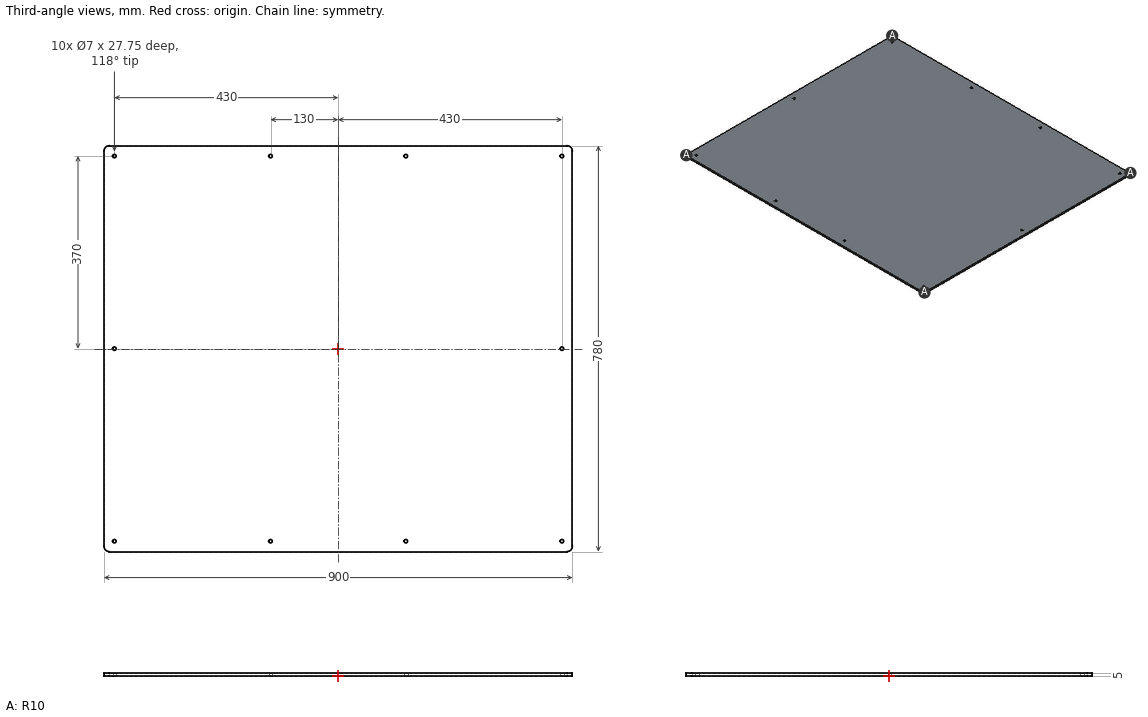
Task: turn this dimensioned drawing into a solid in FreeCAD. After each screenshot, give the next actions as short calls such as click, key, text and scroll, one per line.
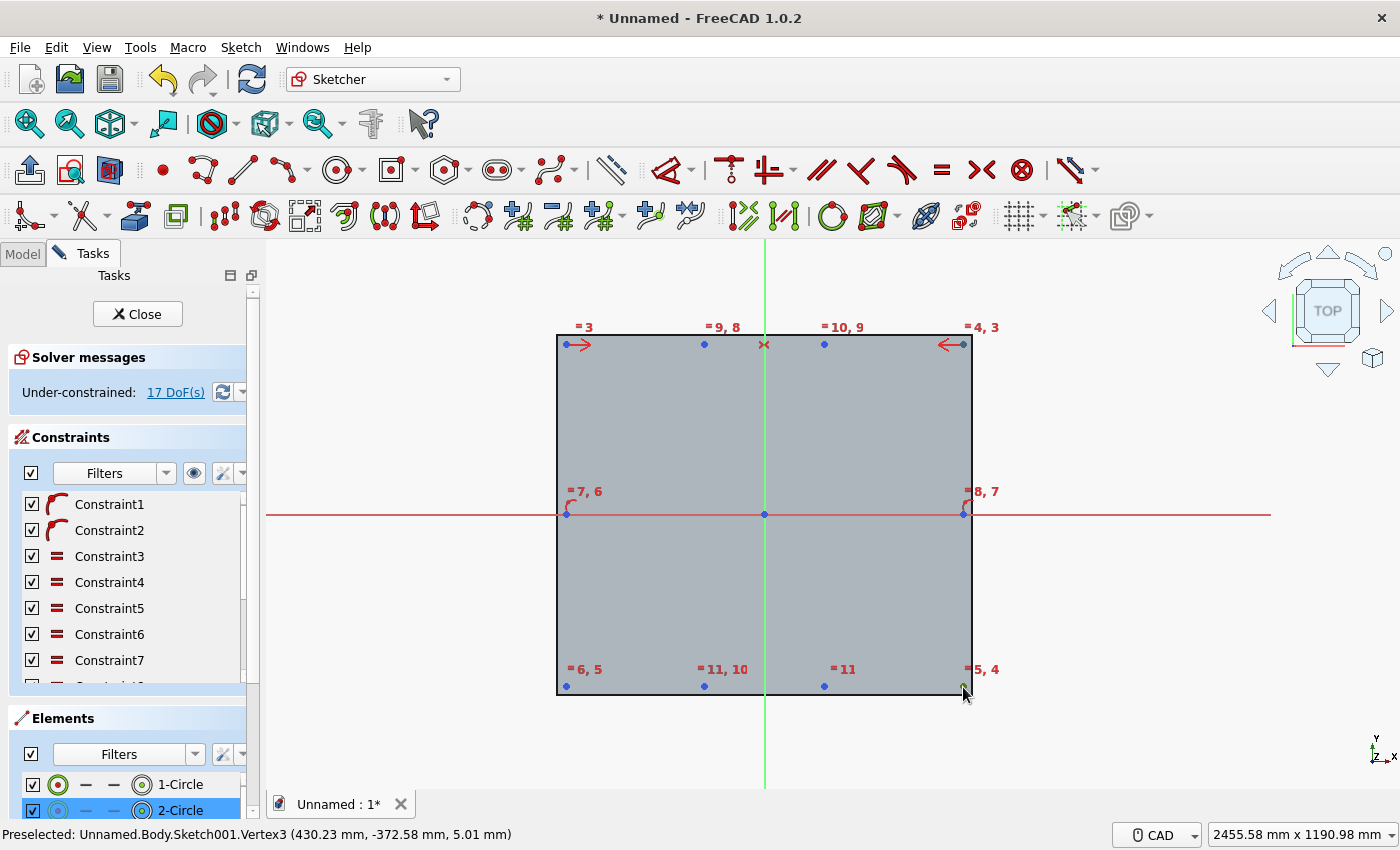
click(361, 515)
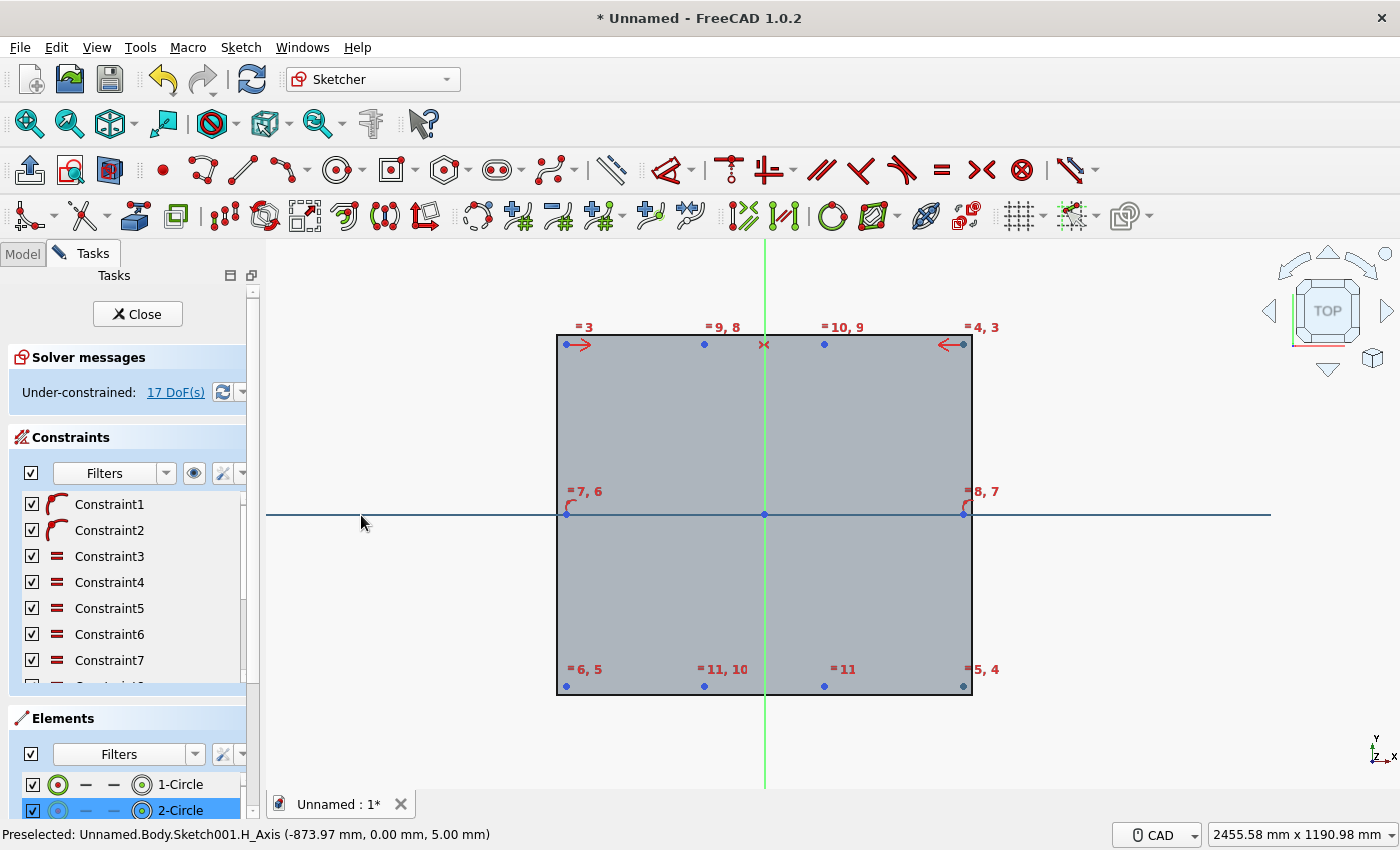
key(s)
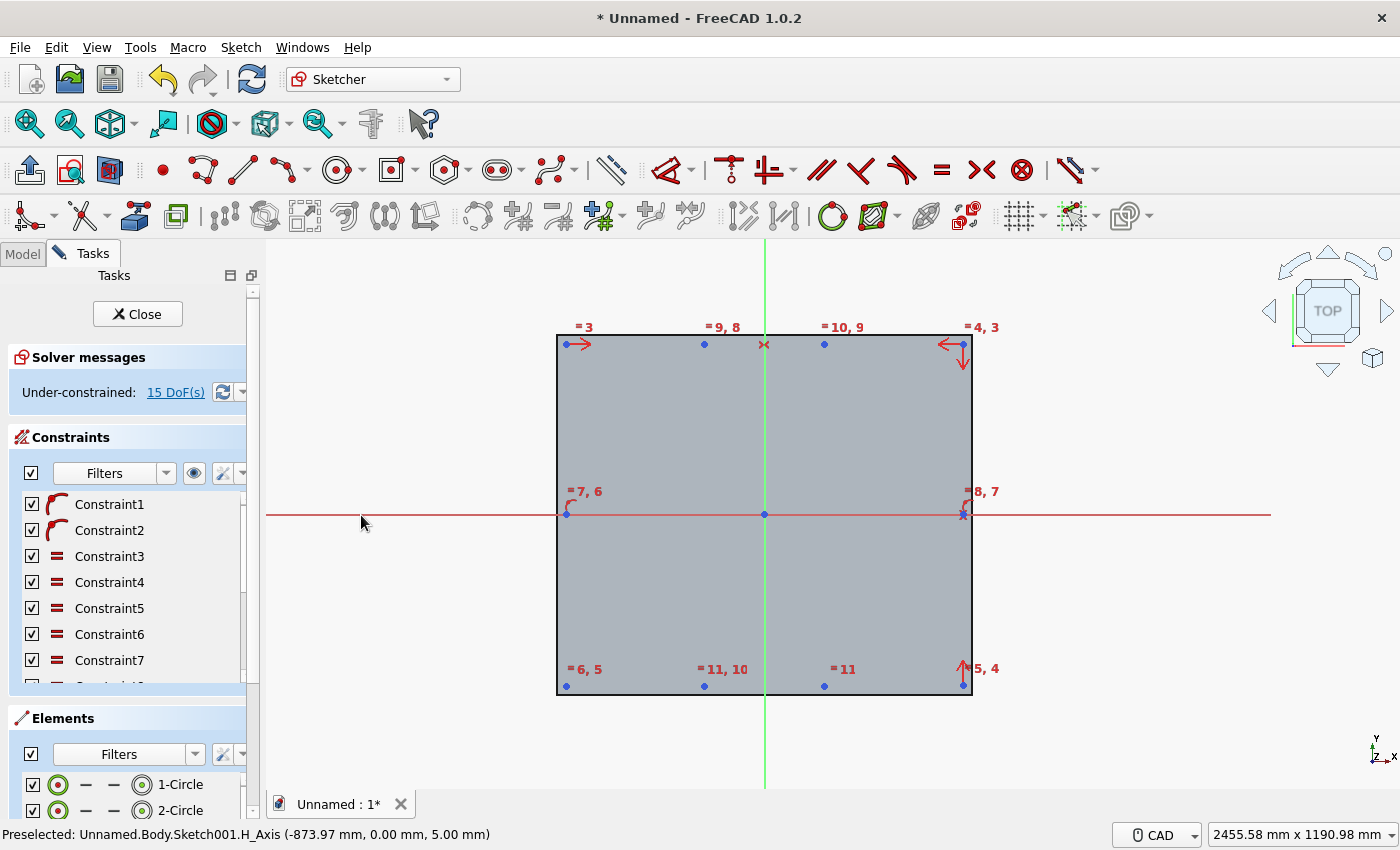
click(566, 344)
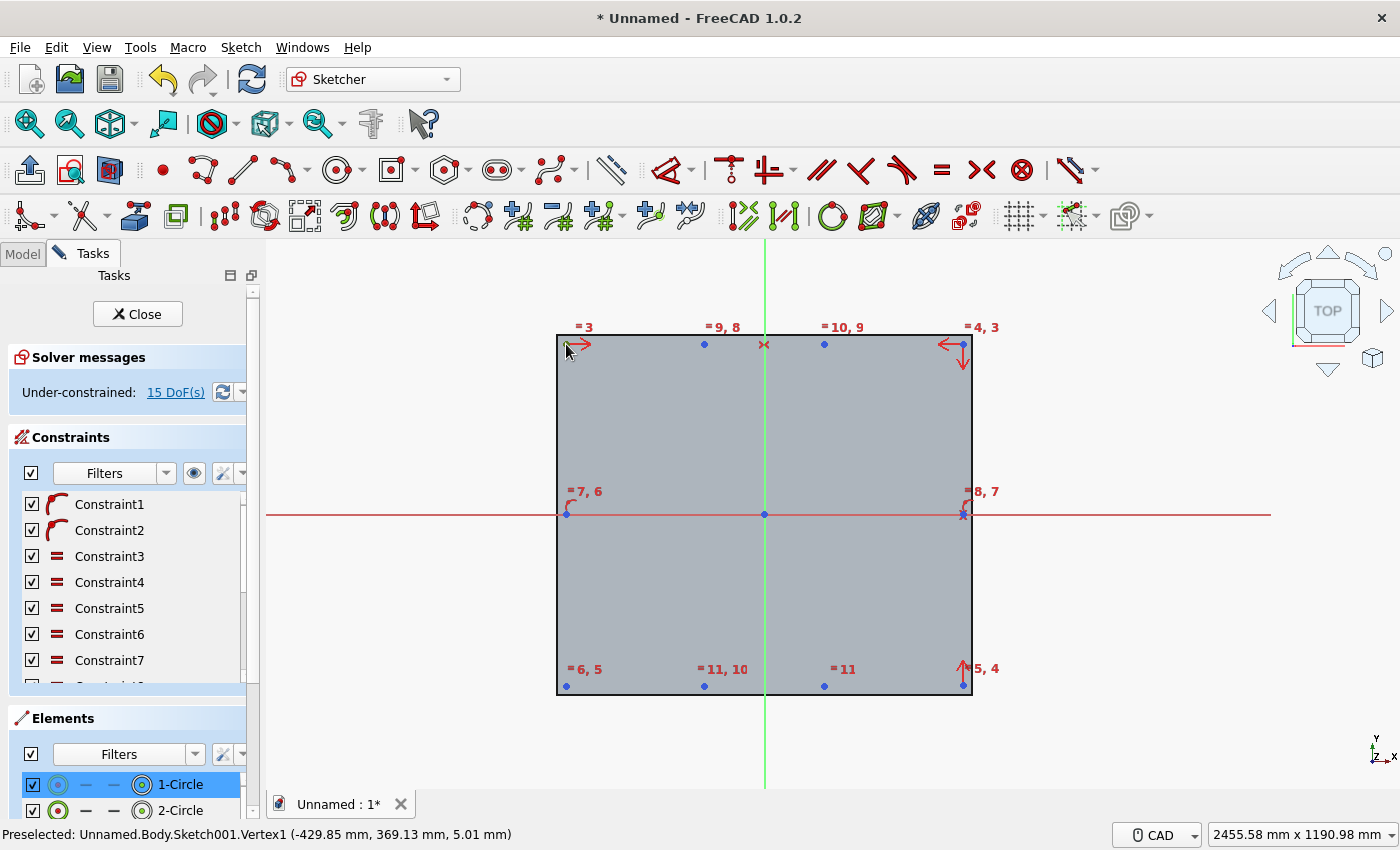
click(566, 687)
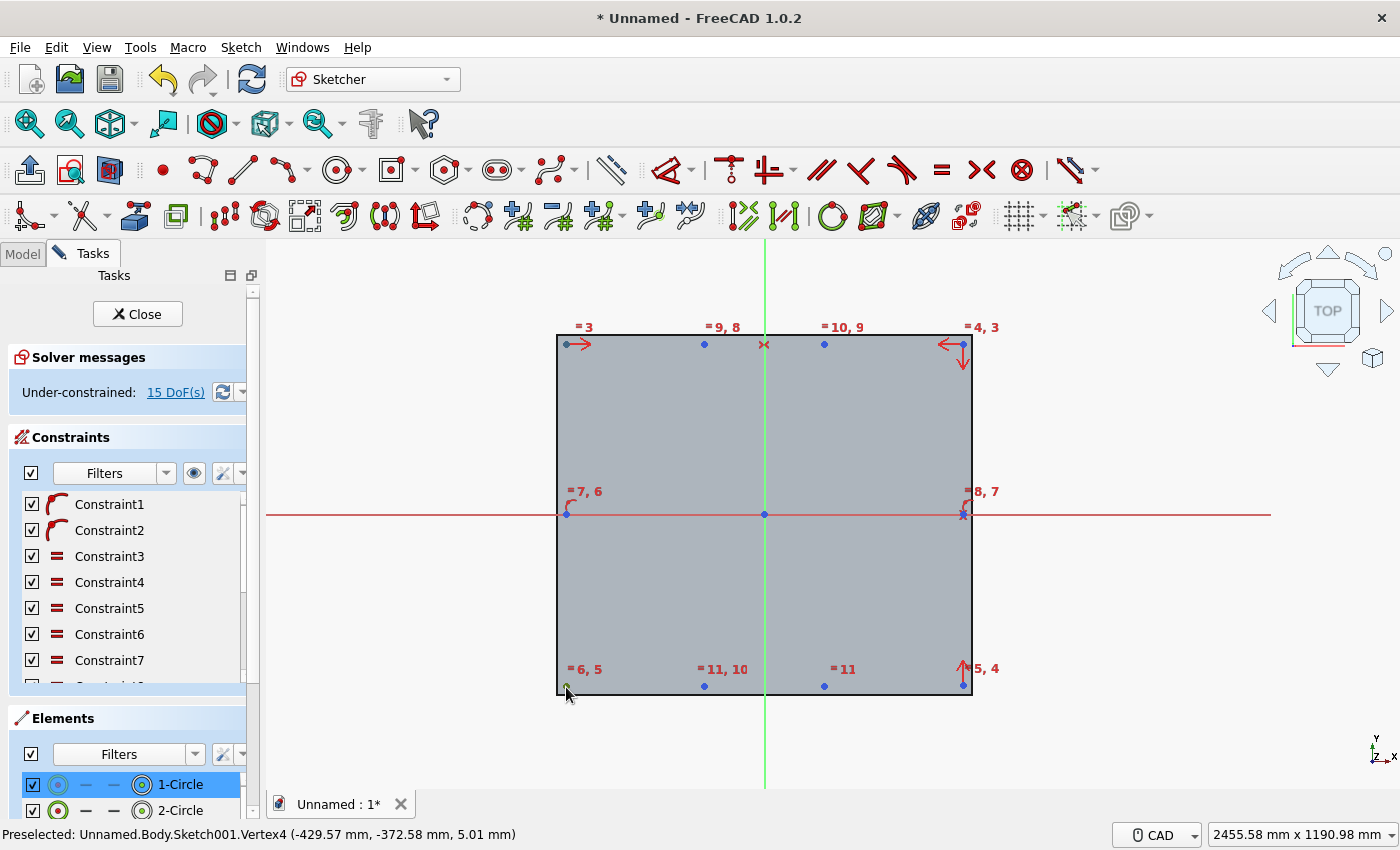
click(361, 515)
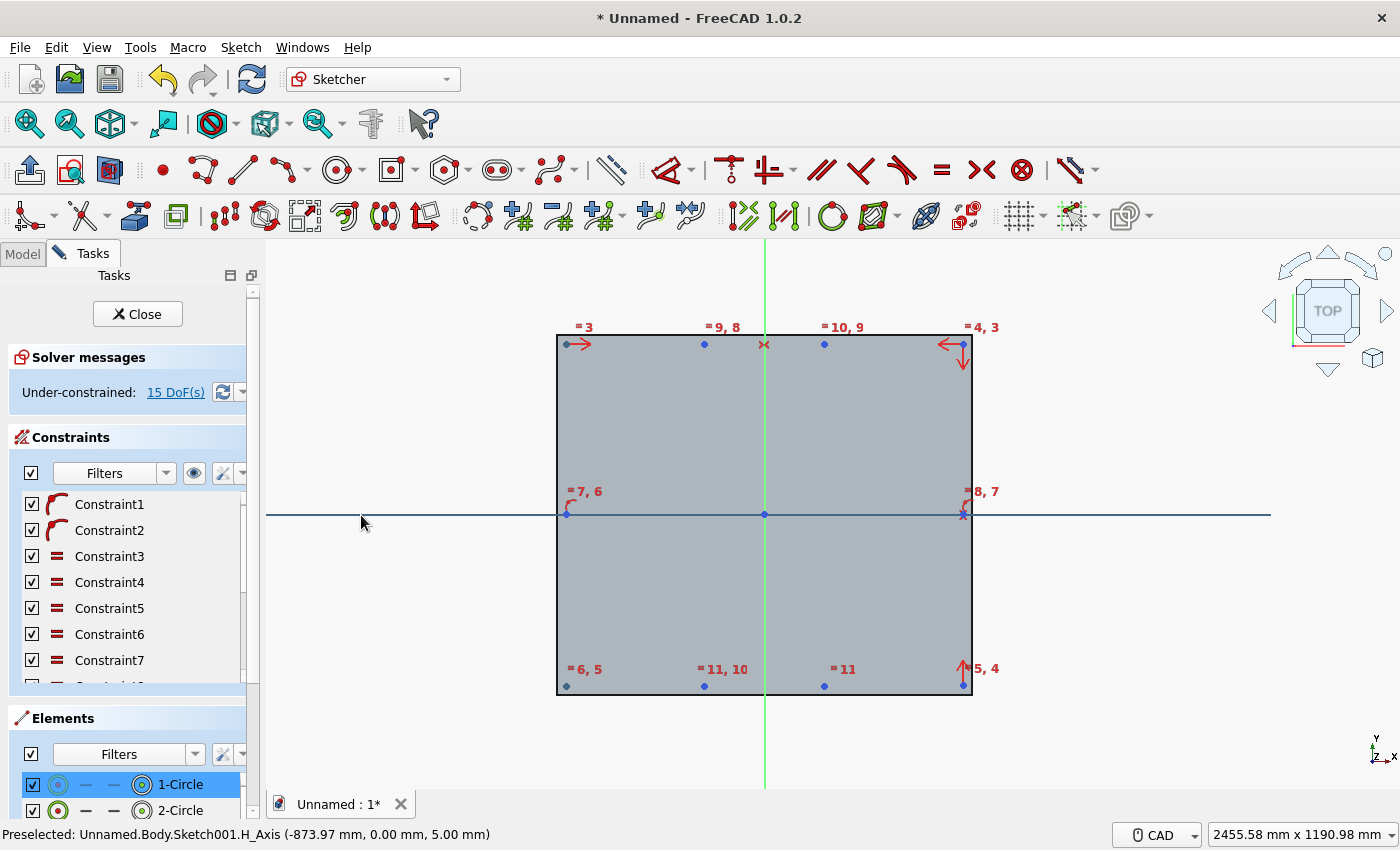
click(982, 170)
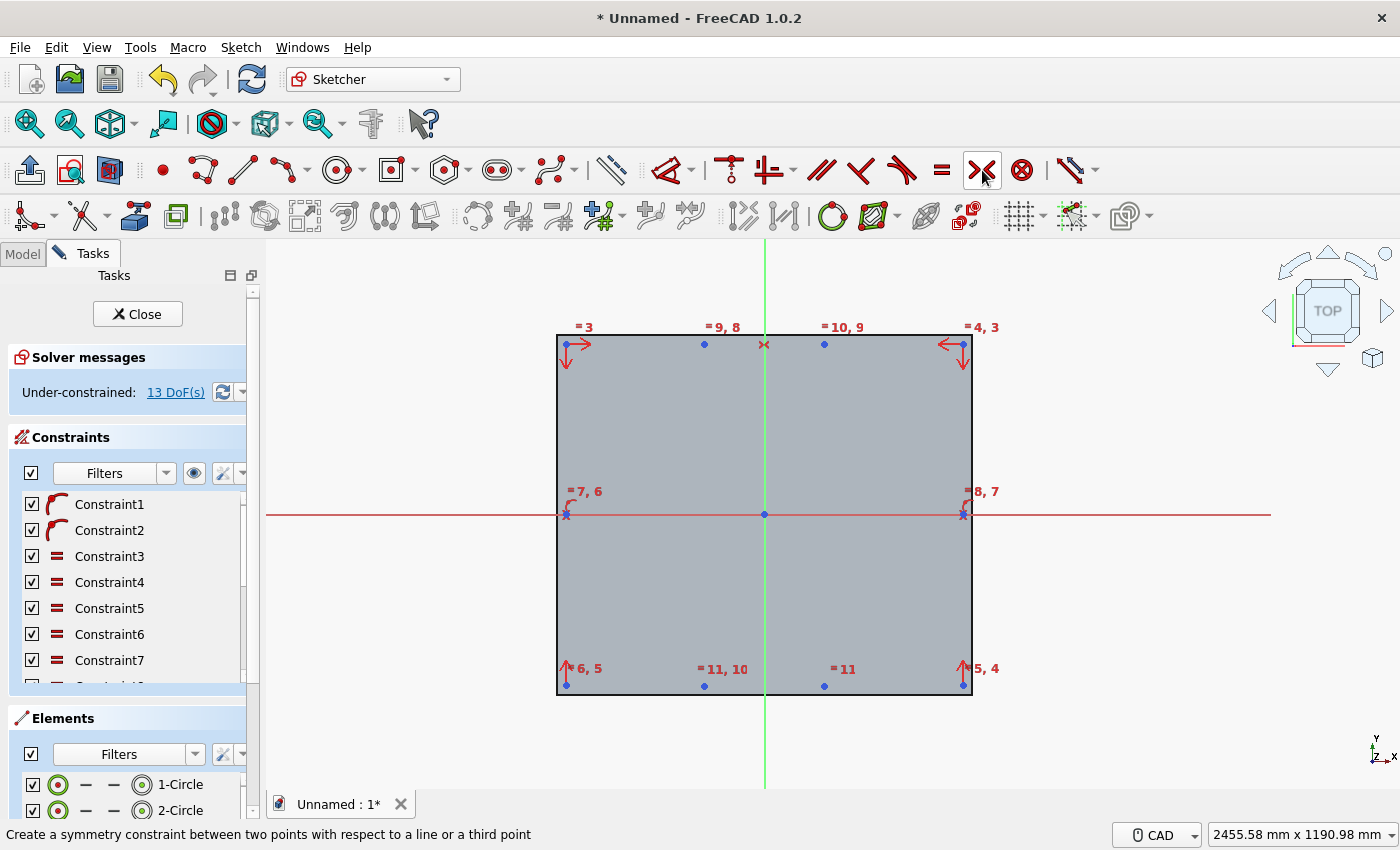
click(704, 345)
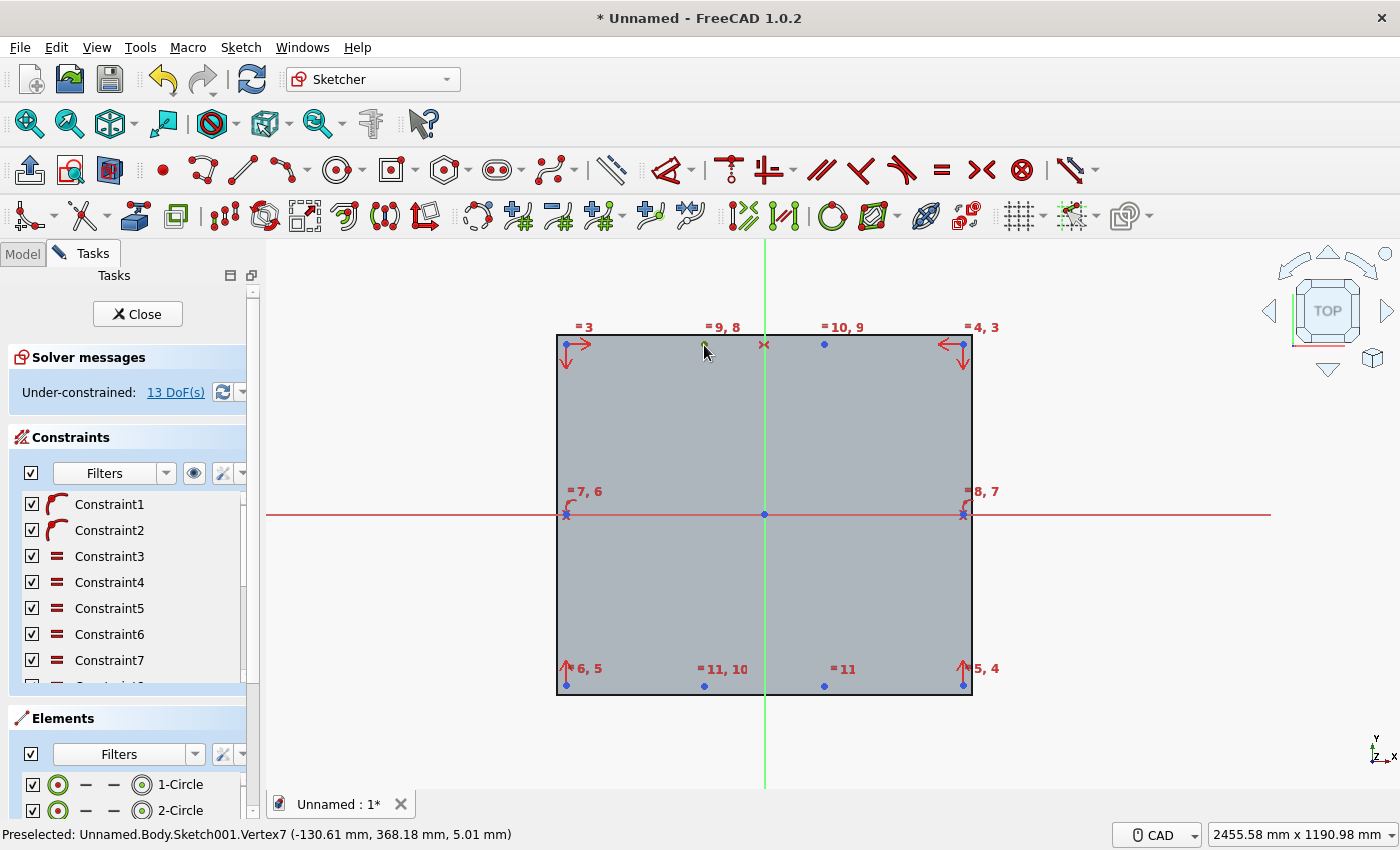
click(824, 345)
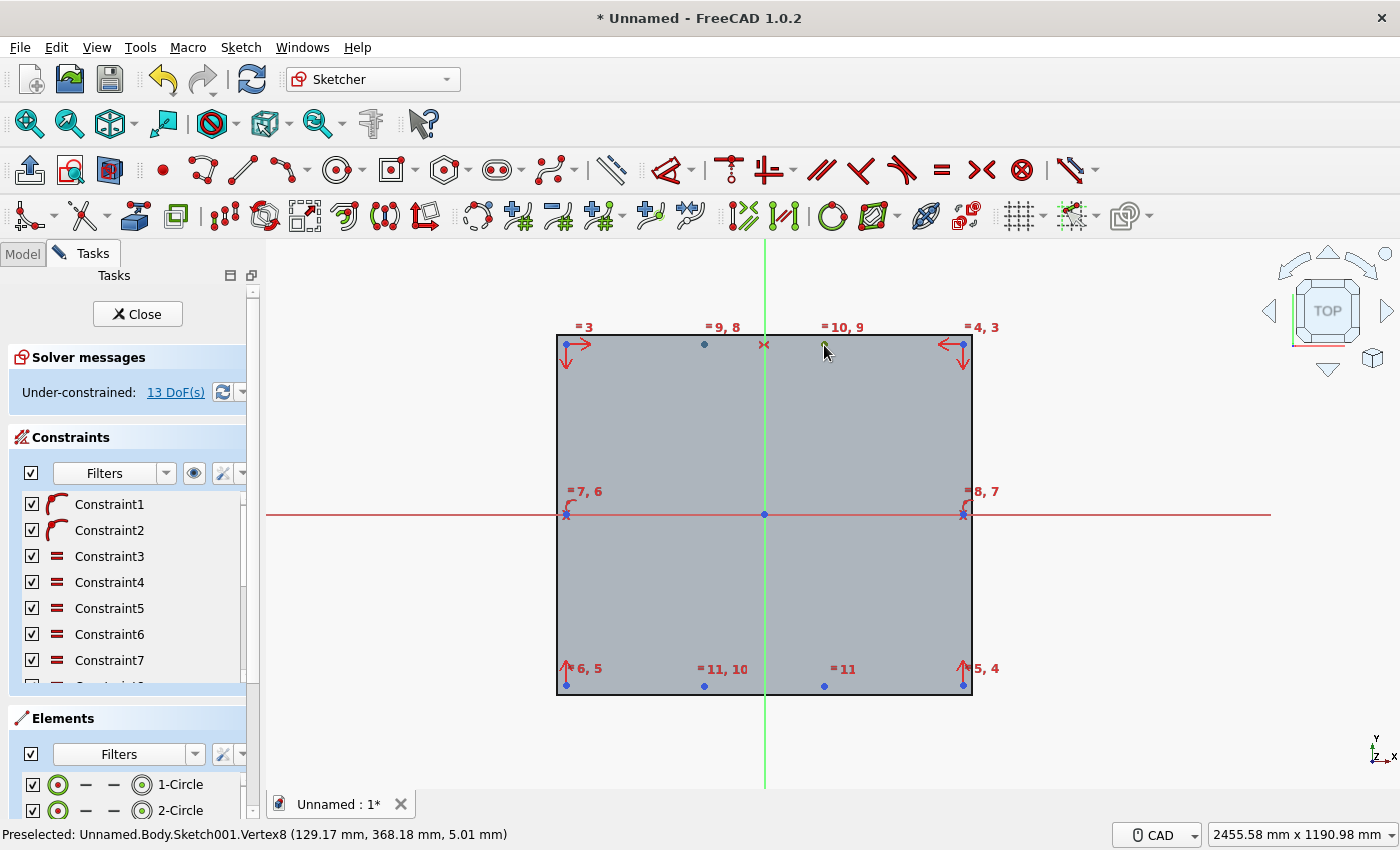
click(765, 726)